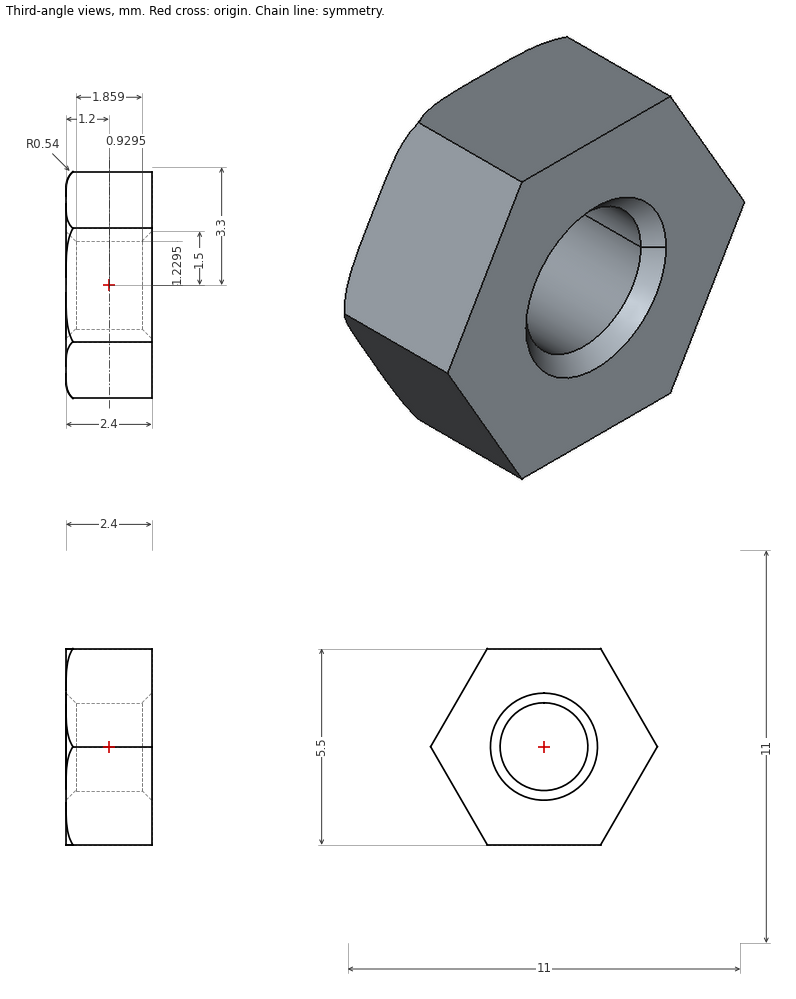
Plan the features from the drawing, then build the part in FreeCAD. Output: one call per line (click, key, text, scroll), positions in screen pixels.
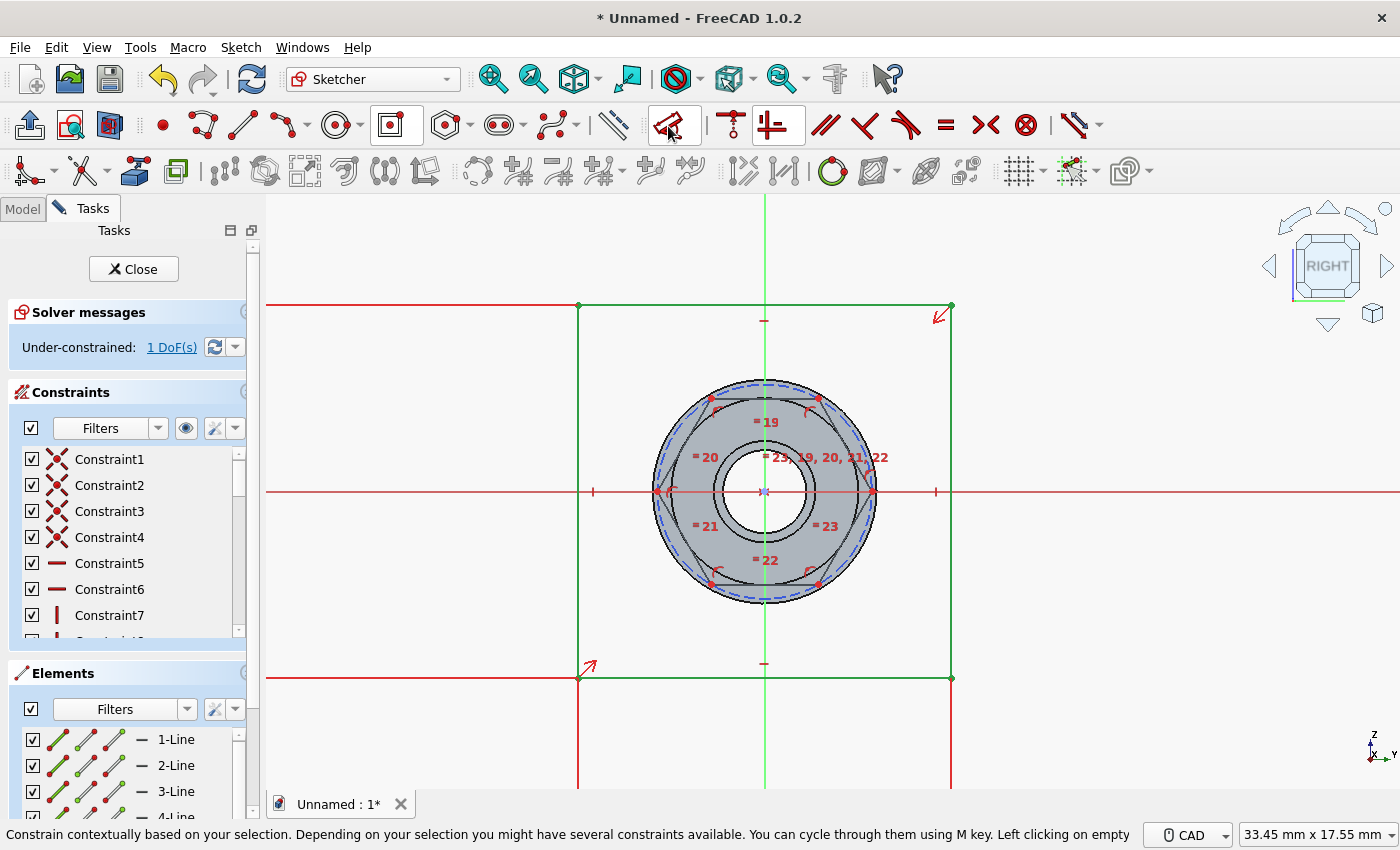
click(711, 585)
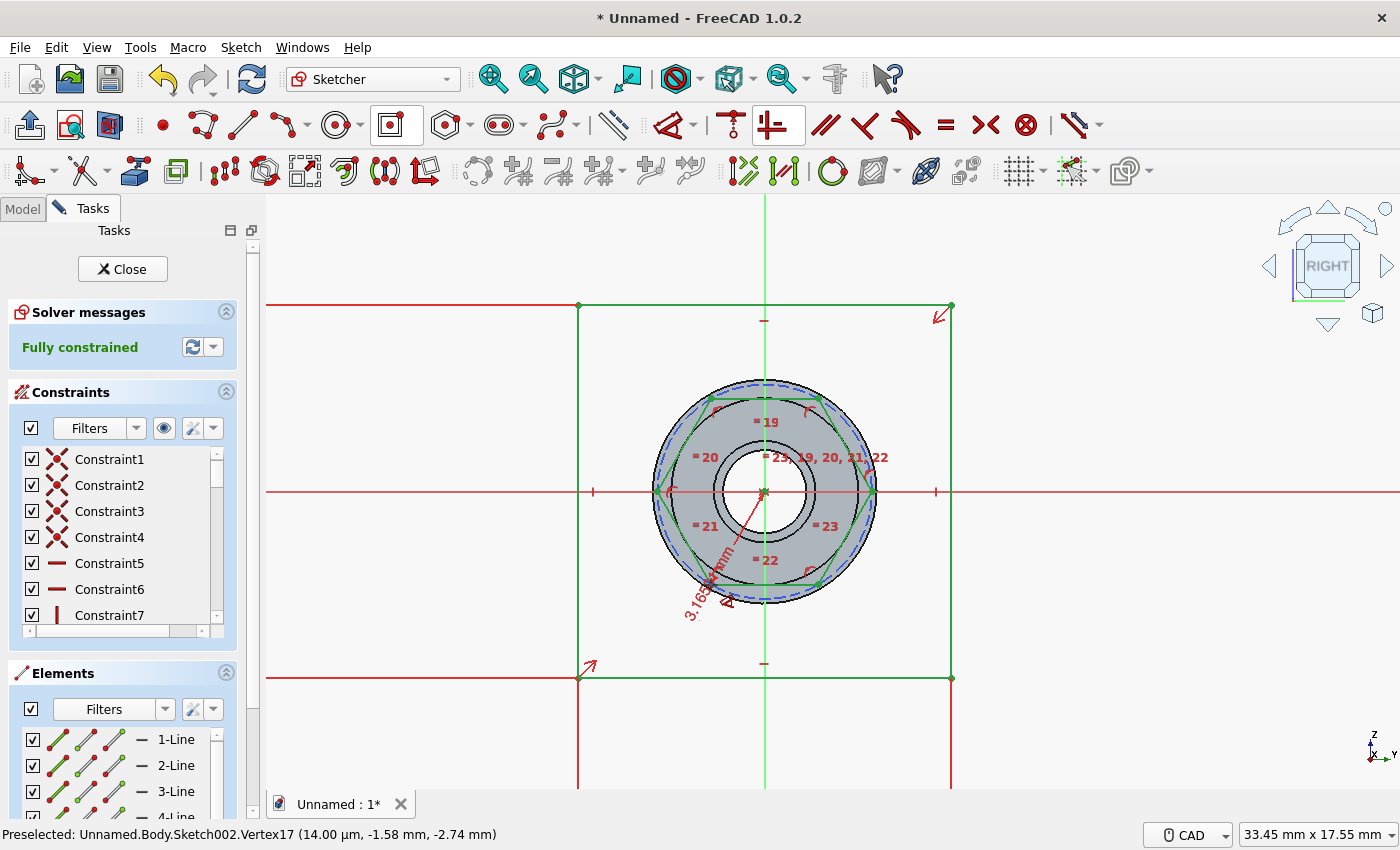
click(818, 399)
click(876, 427)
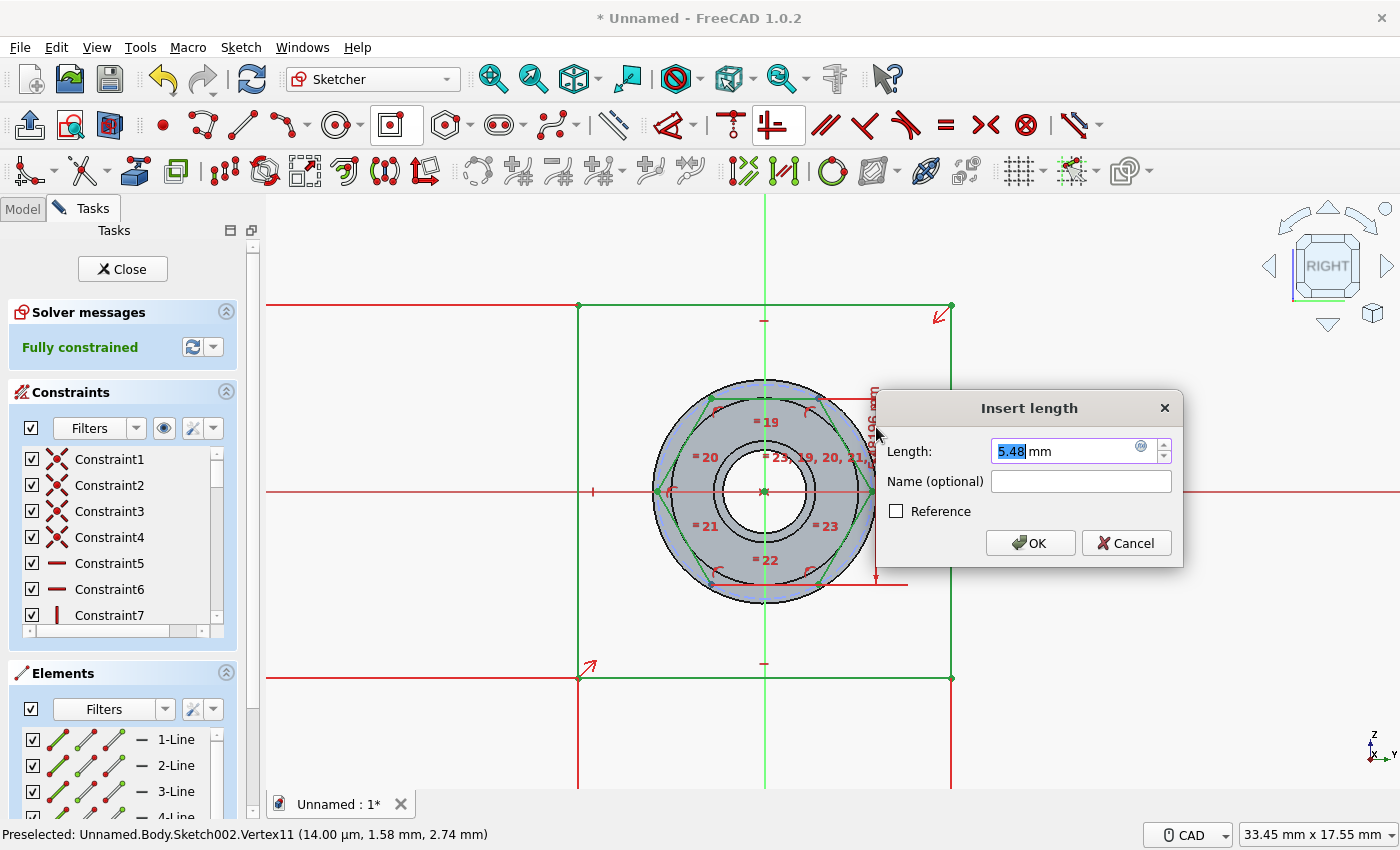
text(5.5)
key(Return)
key(Escape)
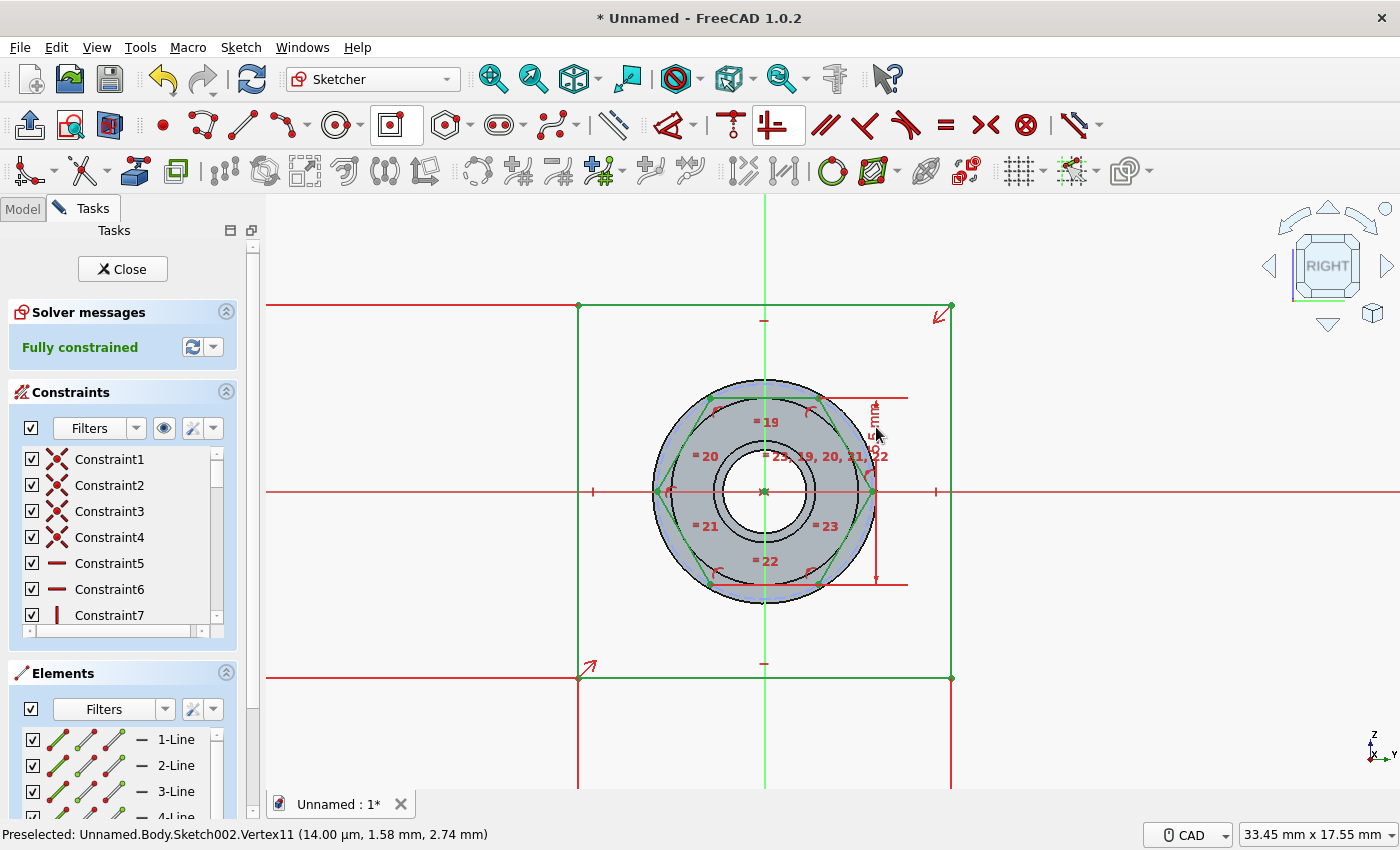
click(123, 269)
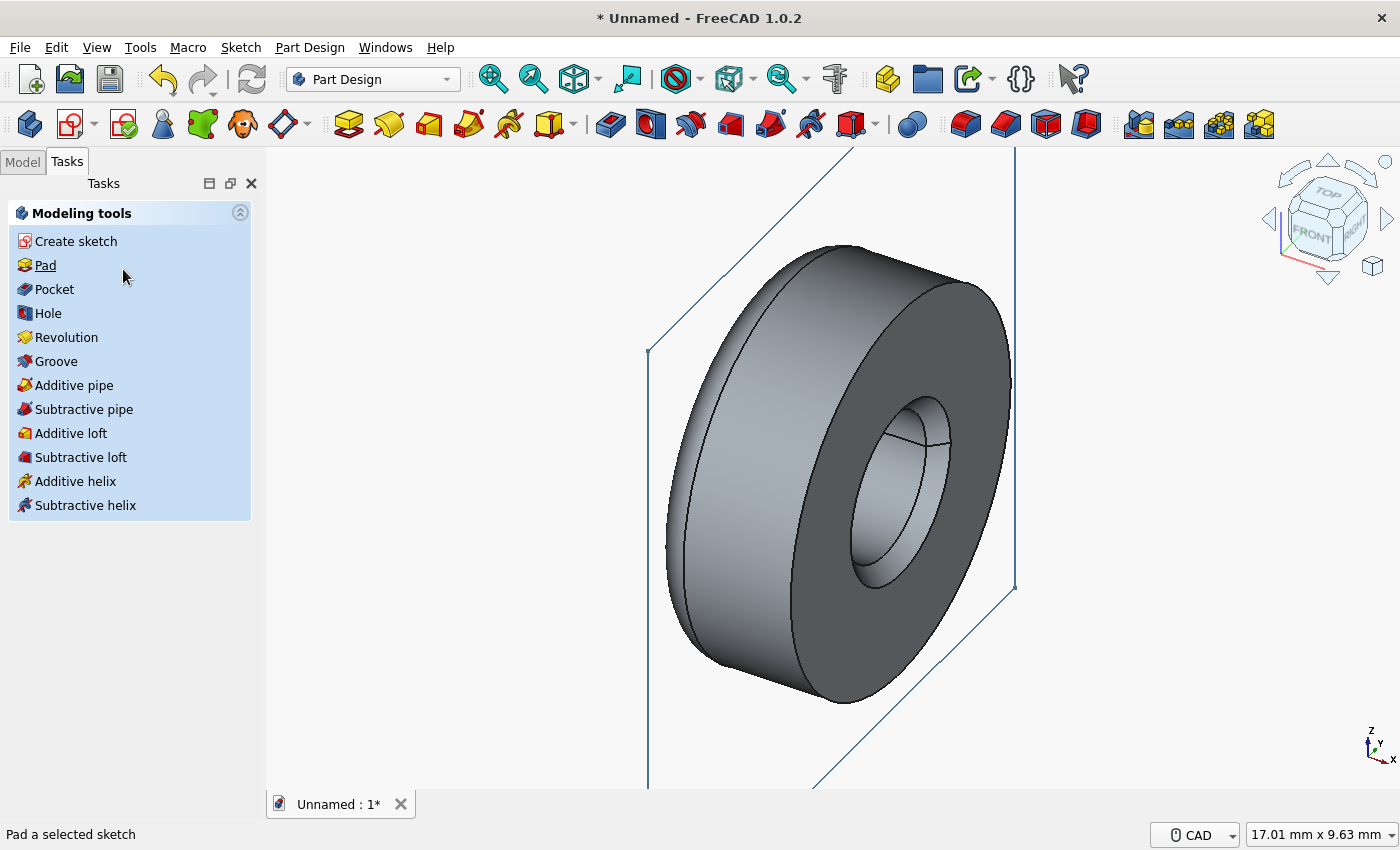
click(612, 124)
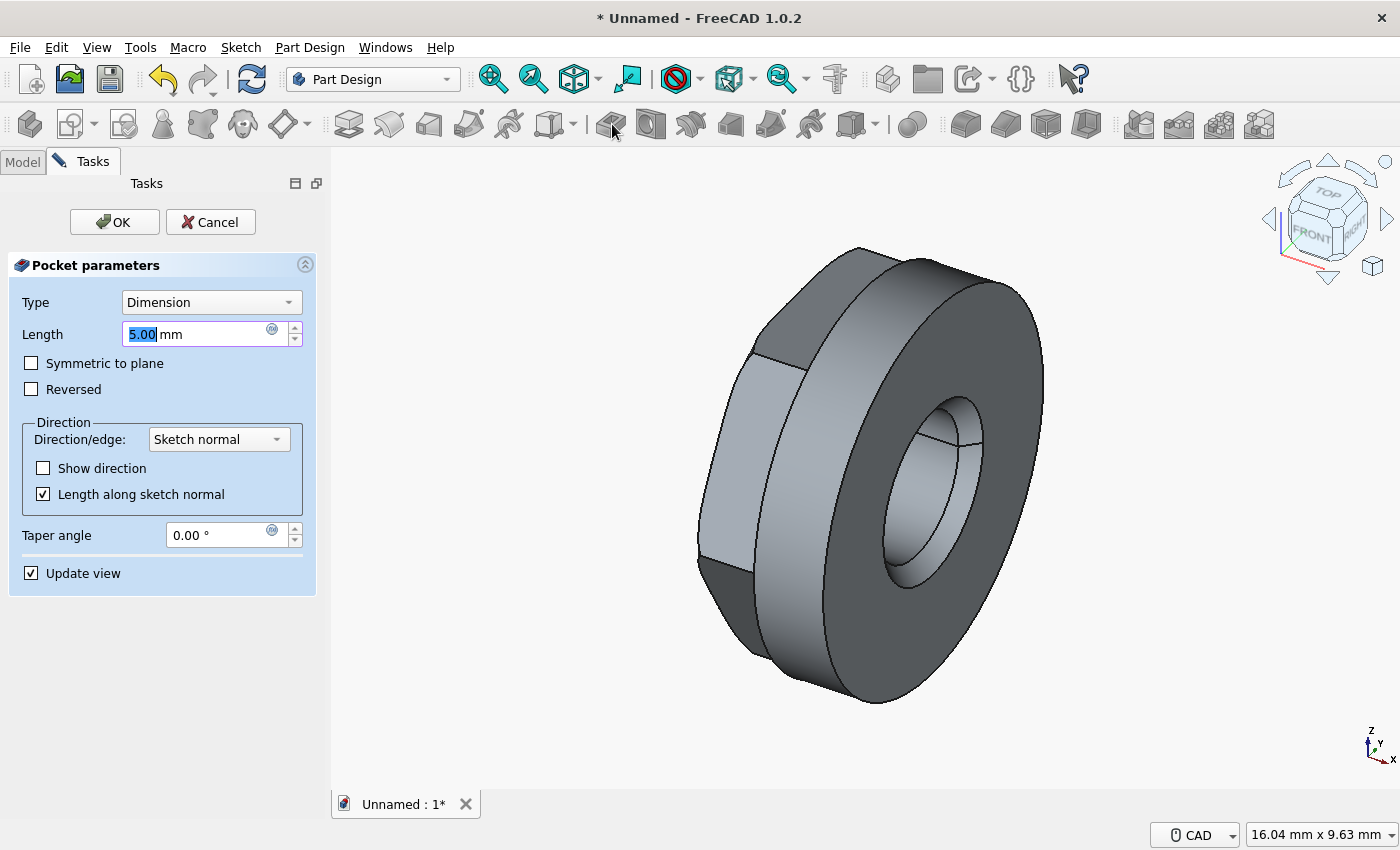
text(2.4)
key(Tab)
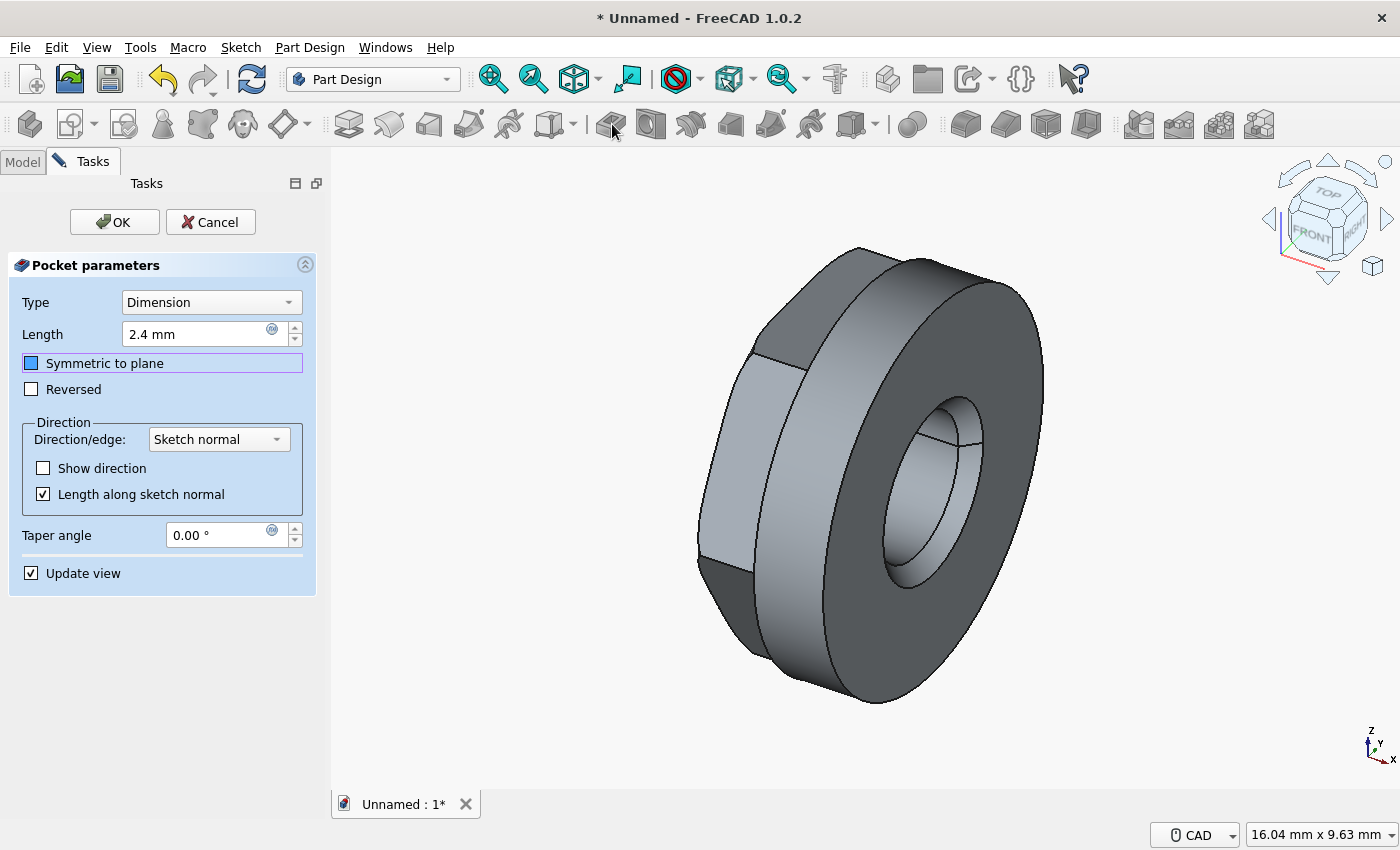
click(30, 363)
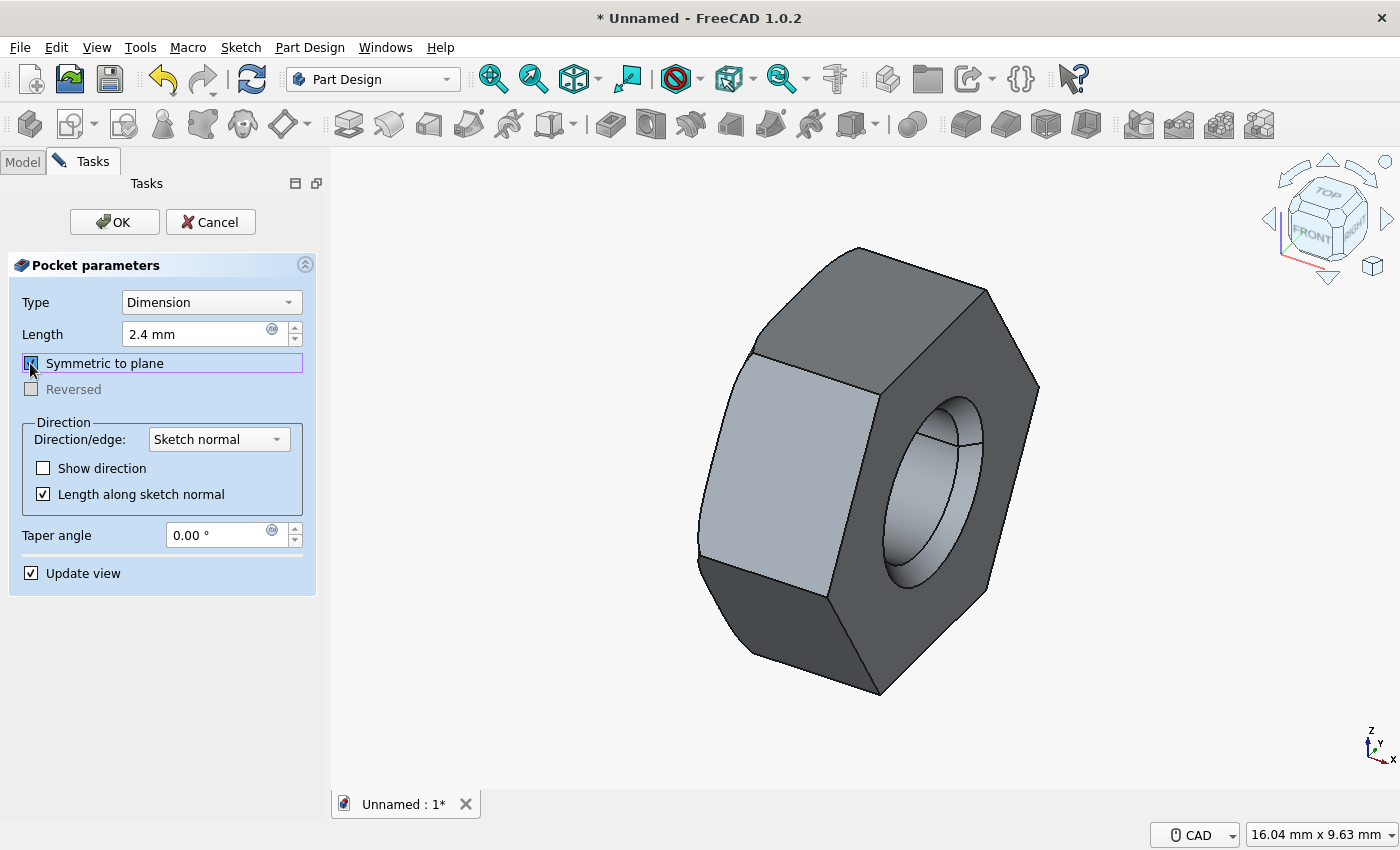
click(115, 222)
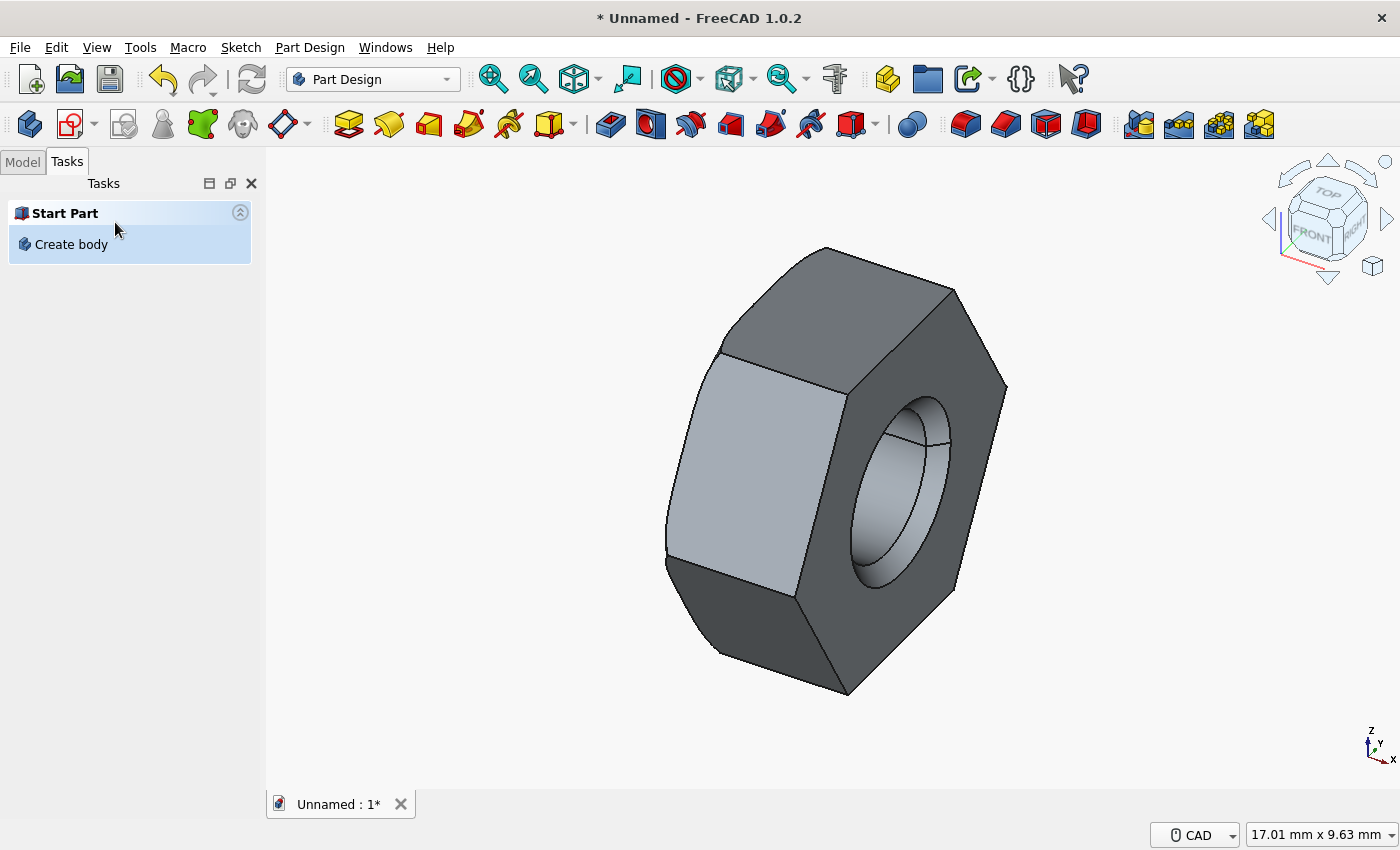
key(0)